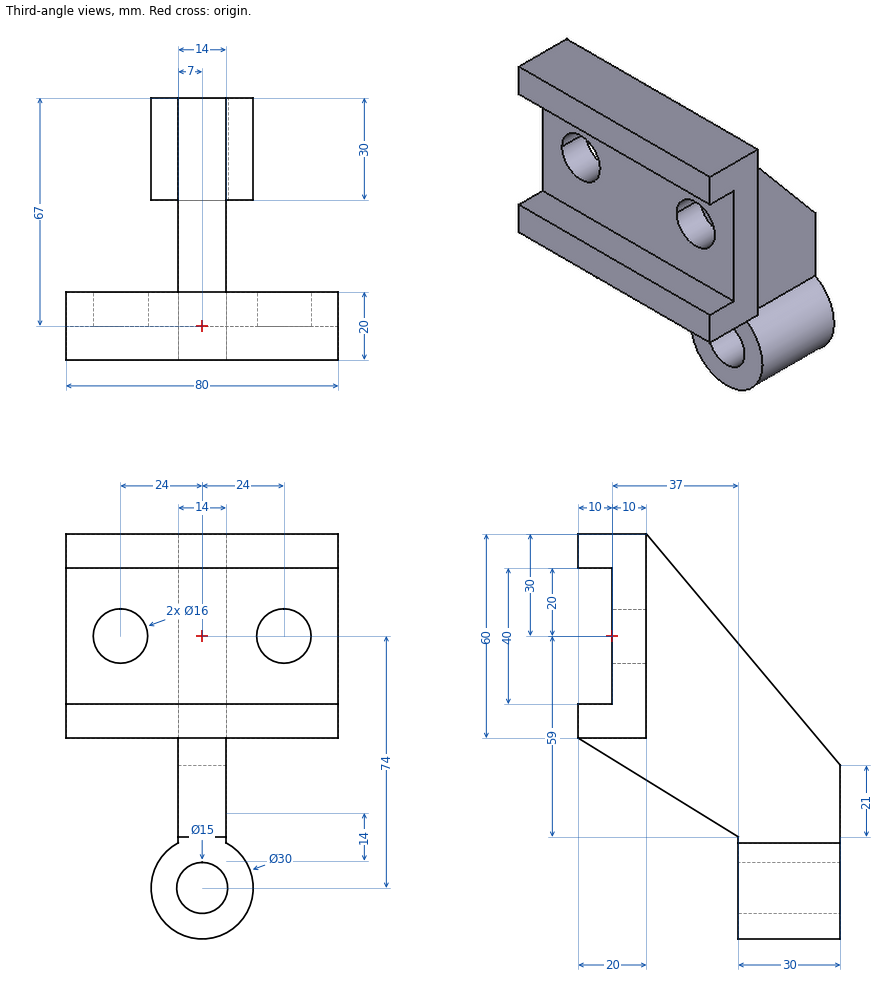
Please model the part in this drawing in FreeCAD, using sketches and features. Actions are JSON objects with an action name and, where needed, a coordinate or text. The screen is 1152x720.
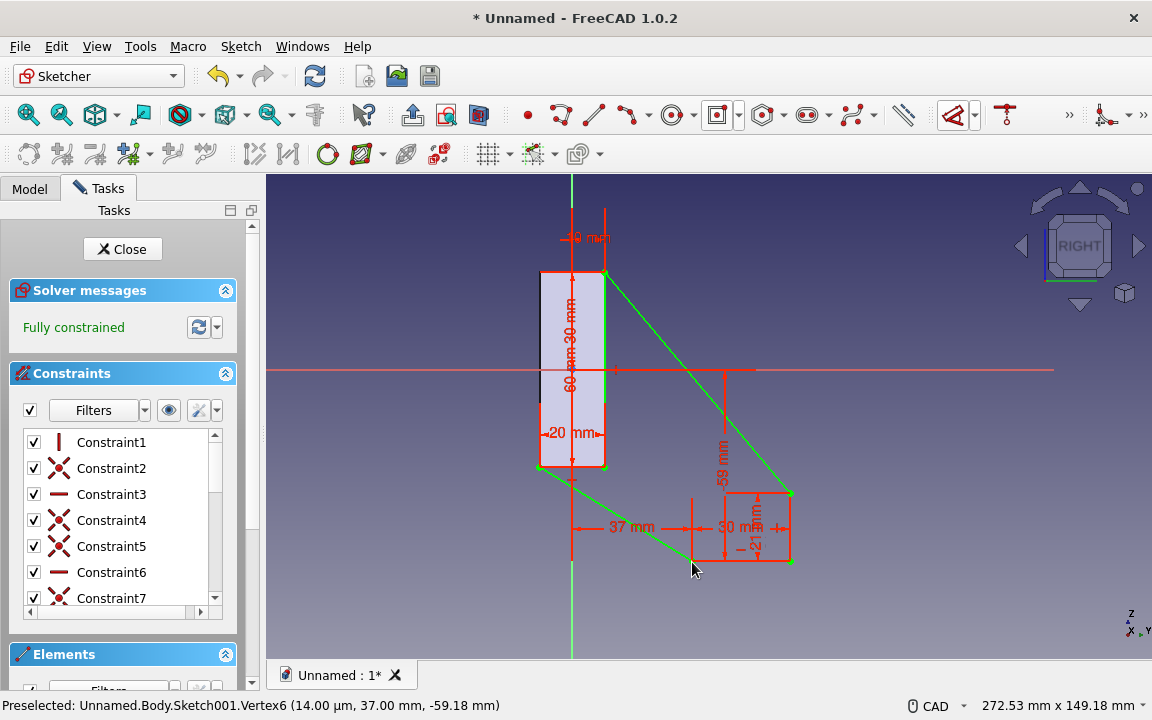
{"action": "left_click", "coordinate": [123, 249]}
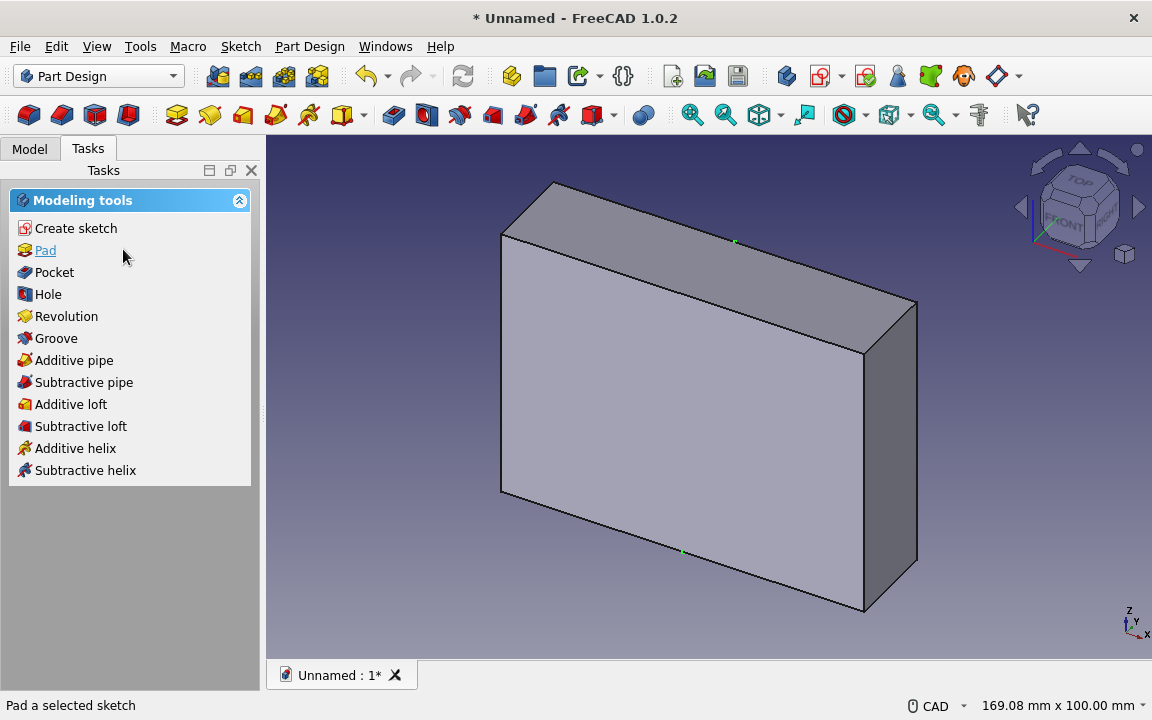
{"action": "left_click", "coordinate": [177, 116]}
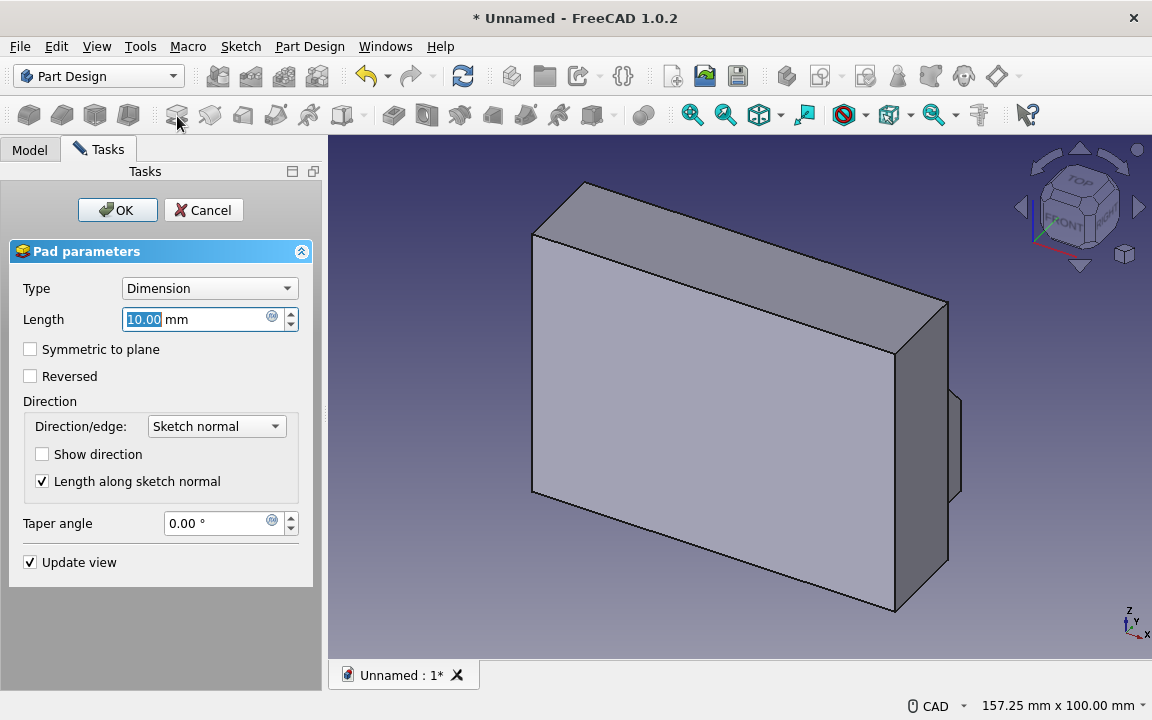
{"action": "type", "text": "14"}
{"action": "key", "text": "Tab"}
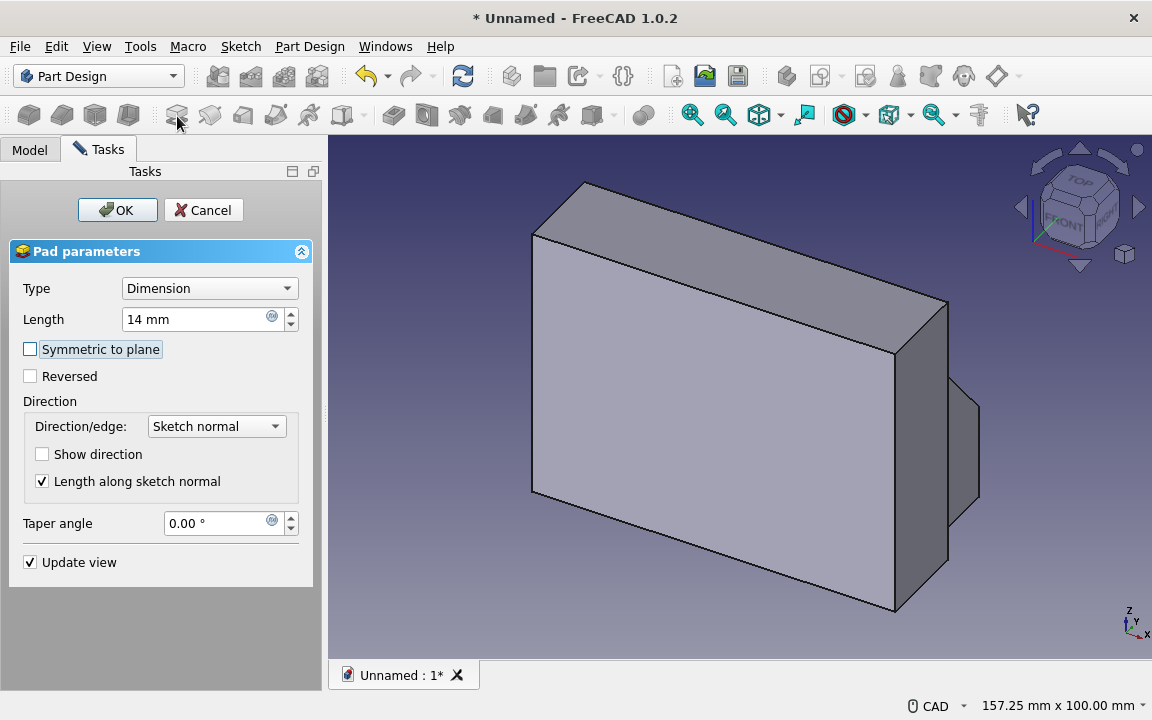
{"action": "left_click", "coordinate": [31, 349]}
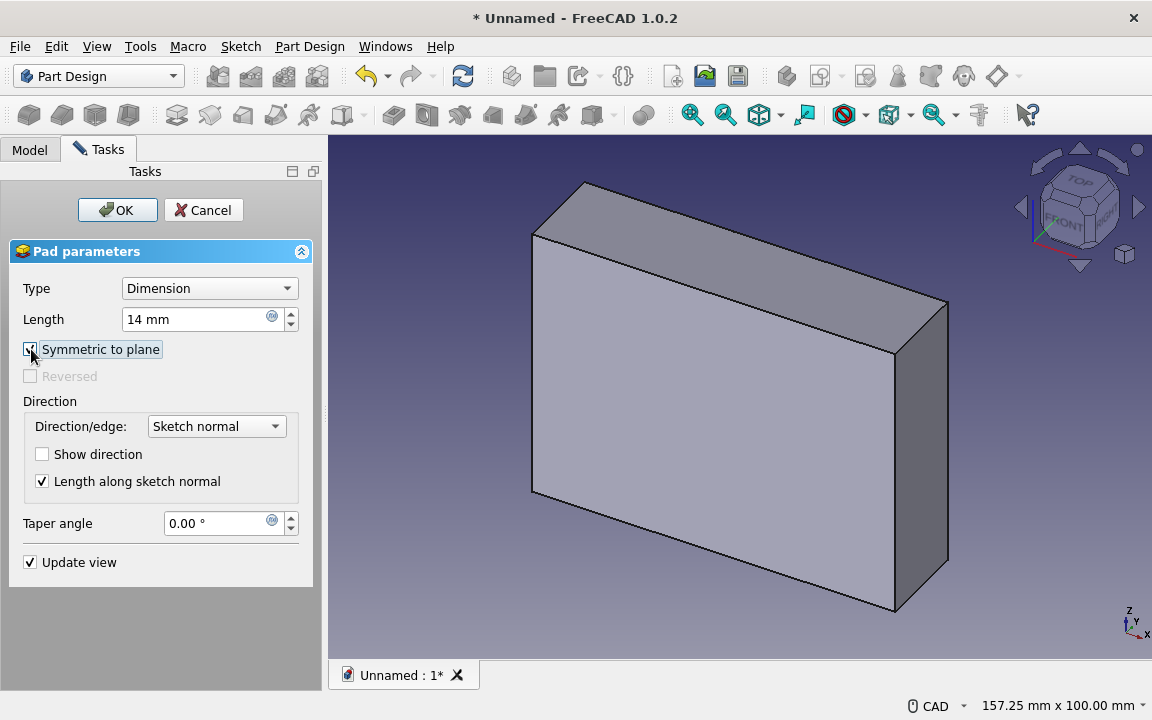
{"action": "left_click", "coordinate": [118, 210]}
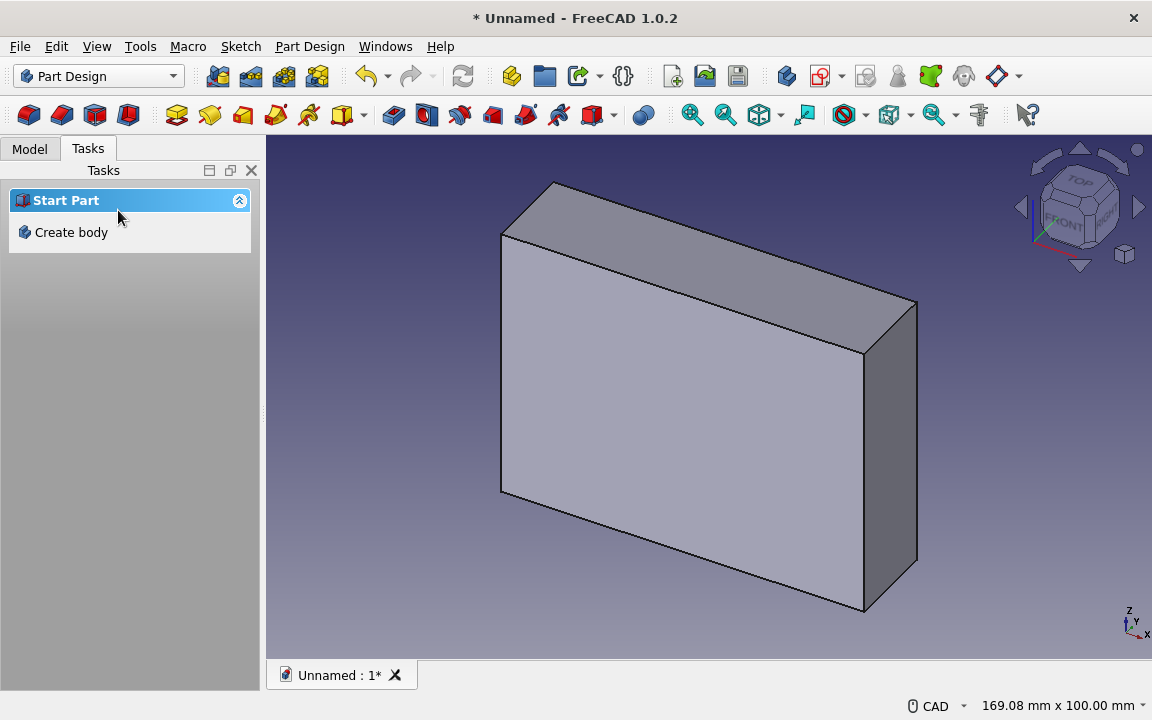
{"action": "left_click", "coordinate": [693, 116]}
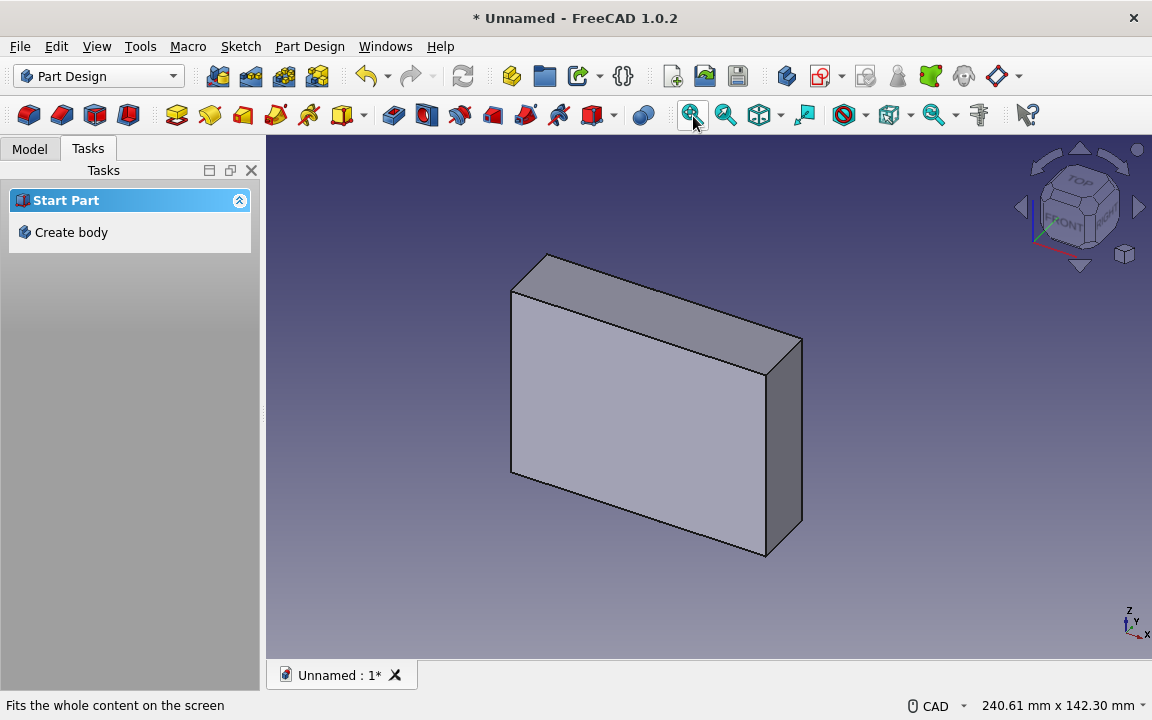
{"action": "left_click", "coordinate": [787, 76]}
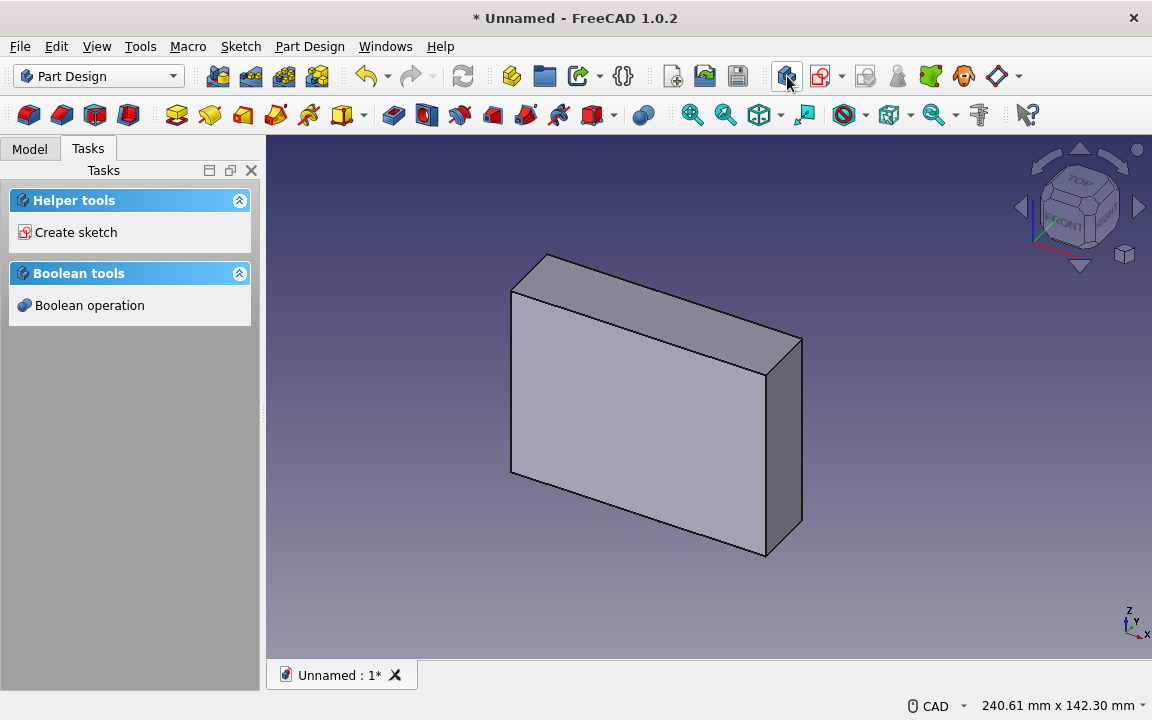
{"action": "left_click", "coordinate": [30, 148]}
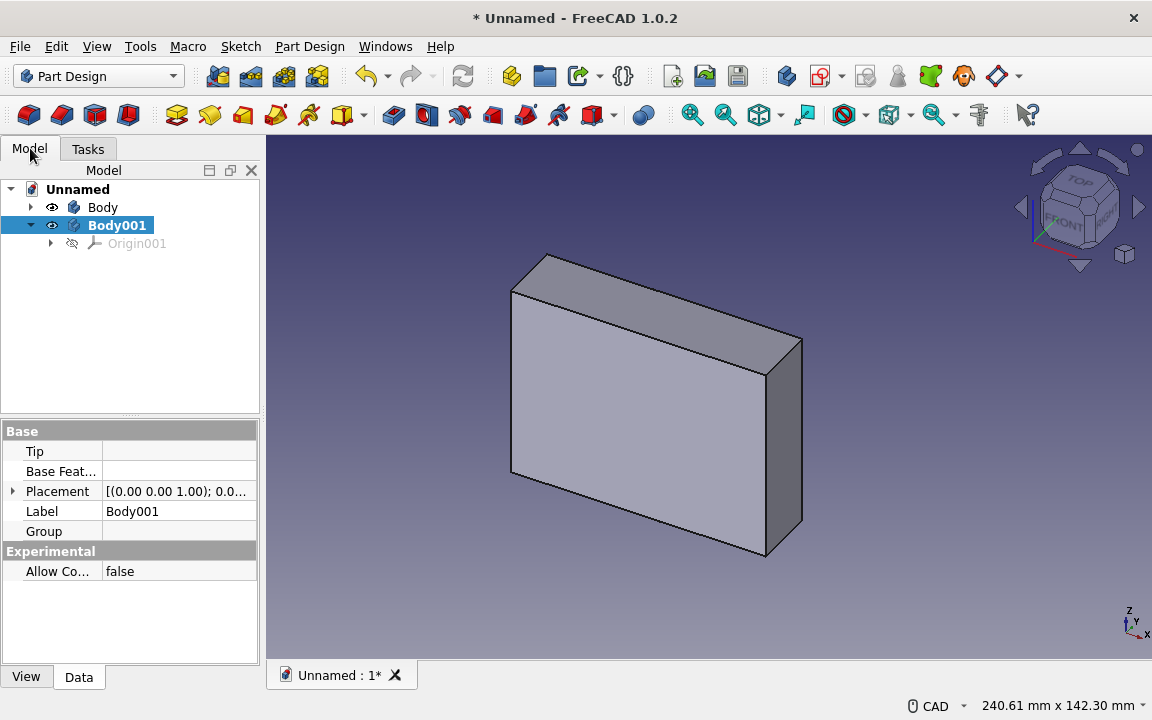
{"action": "left_click", "coordinate": [51, 243]}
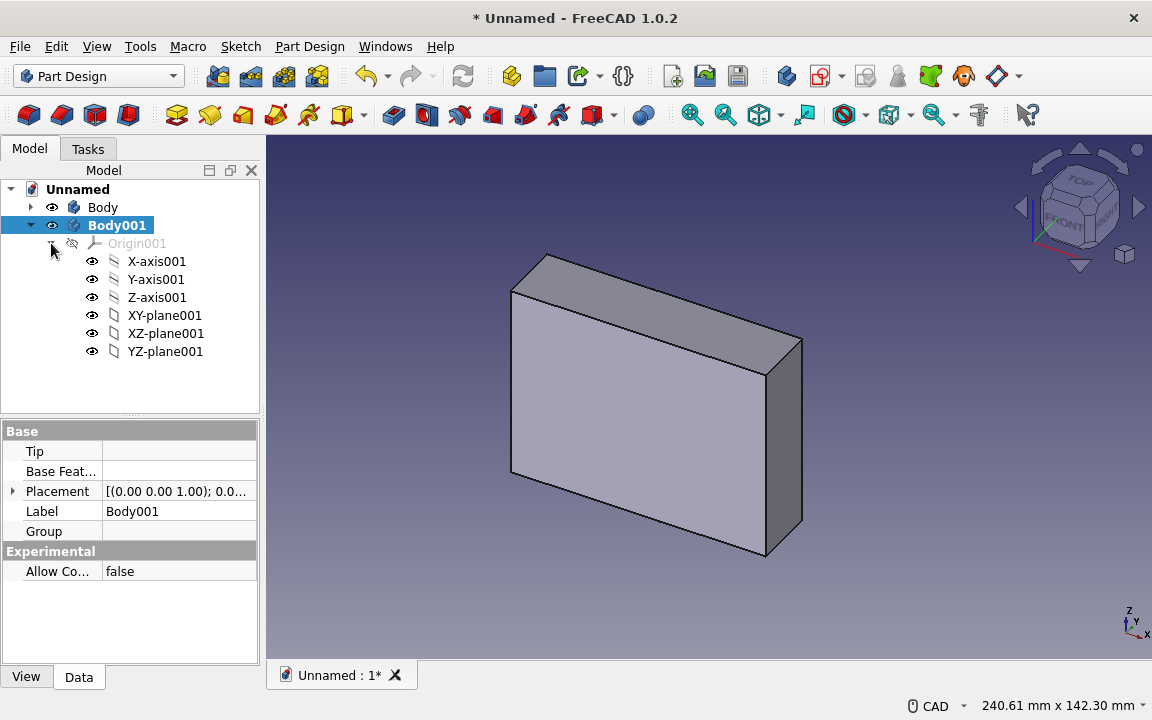
{"action": "left_click", "coordinate": [137, 333]}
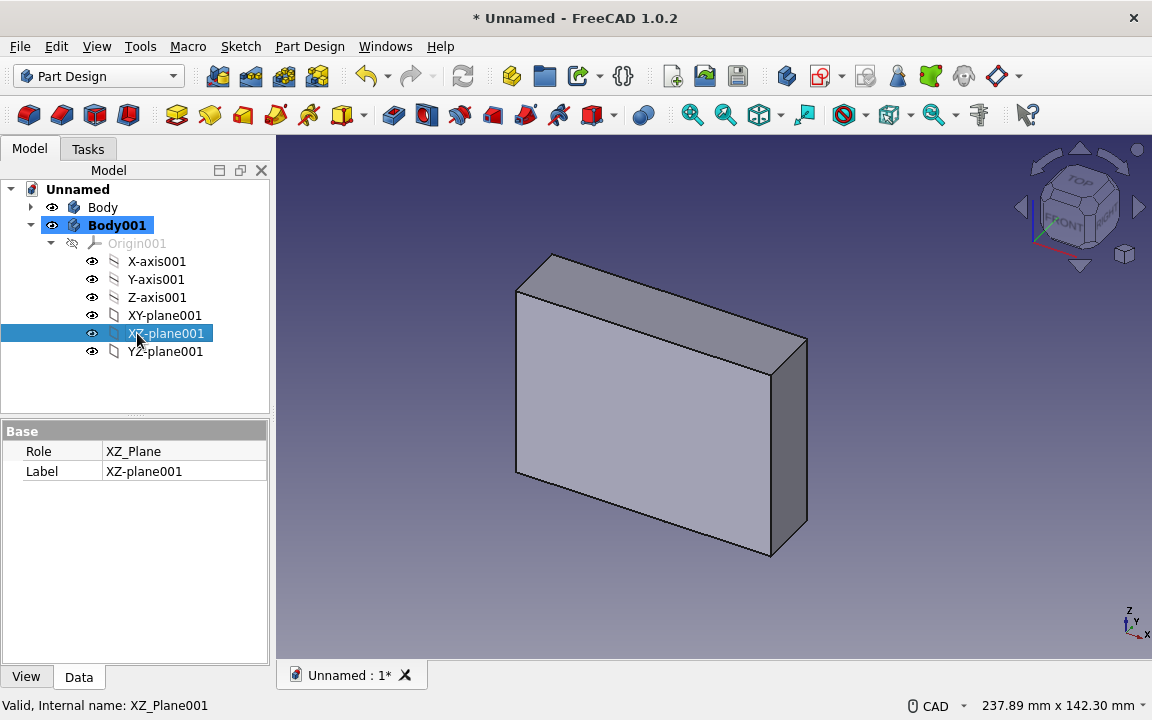
{"action": "left_click", "coordinate": [996, 76]}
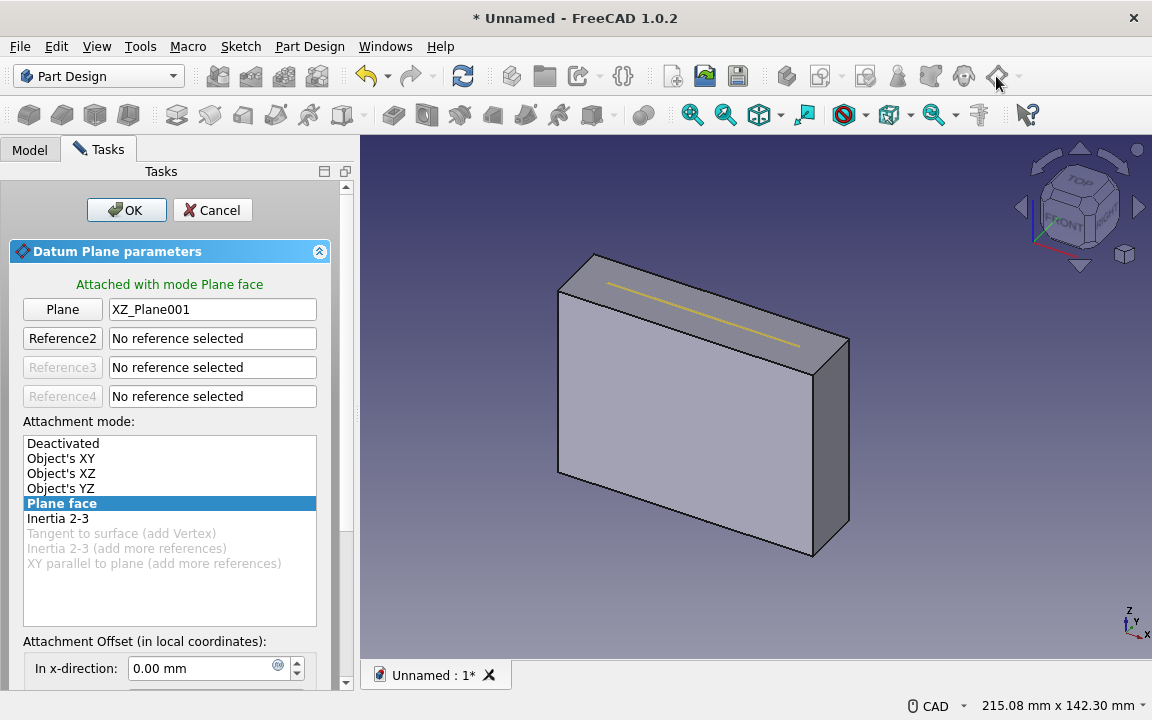
{"action": "scroll", "coordinate": [346, 436], "scroll_direction": "down", "scroll_amount": 2}